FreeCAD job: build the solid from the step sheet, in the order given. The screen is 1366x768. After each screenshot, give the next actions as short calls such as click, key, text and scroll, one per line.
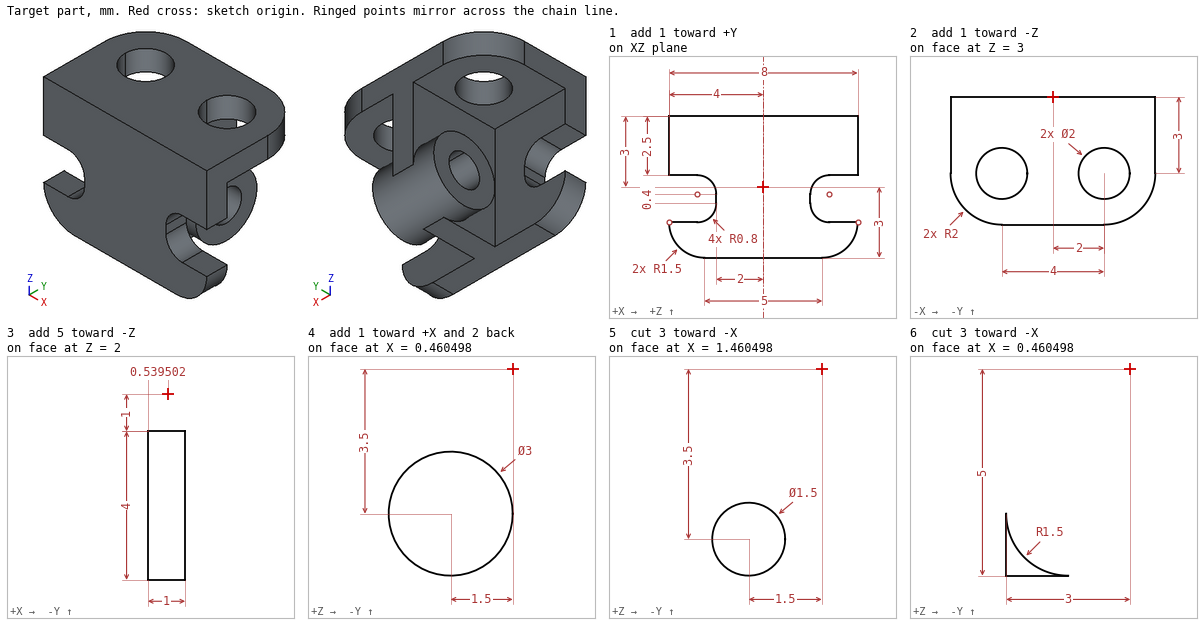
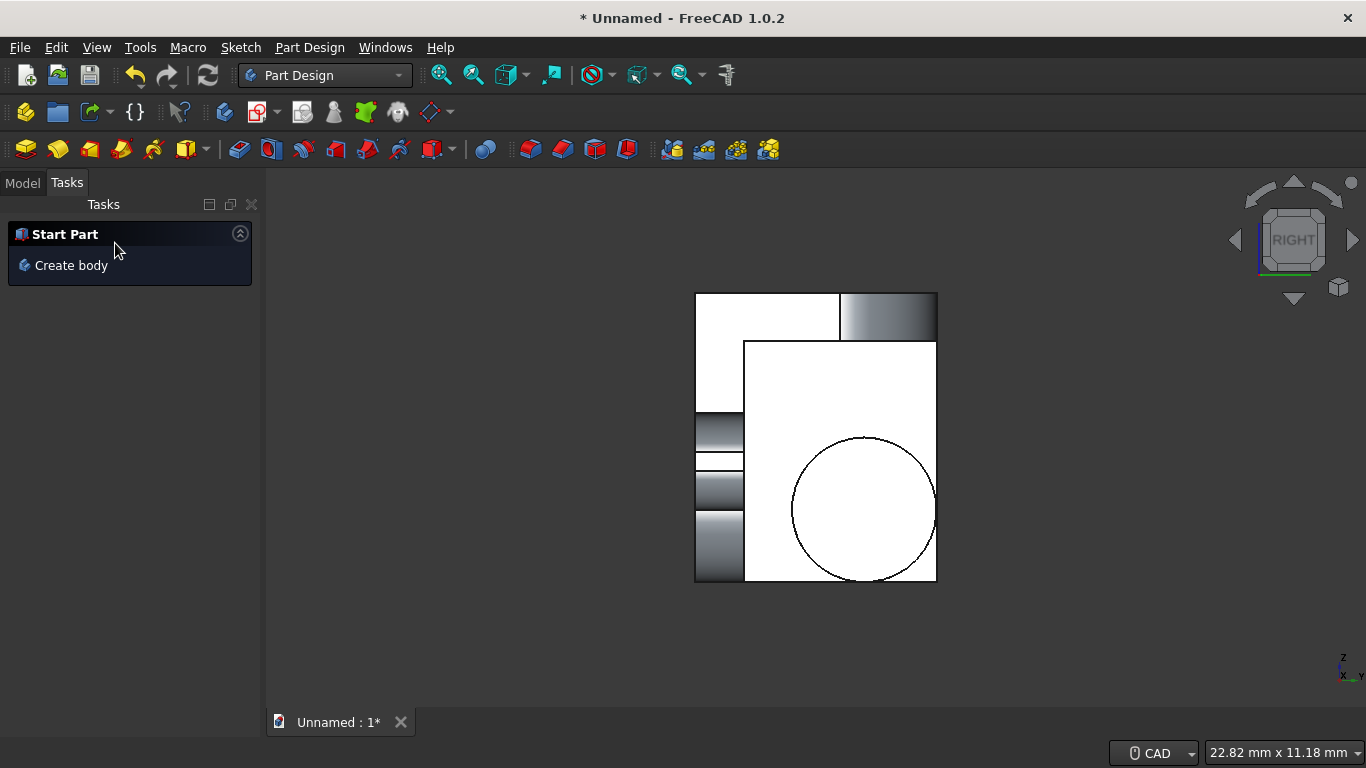
click(864, 509)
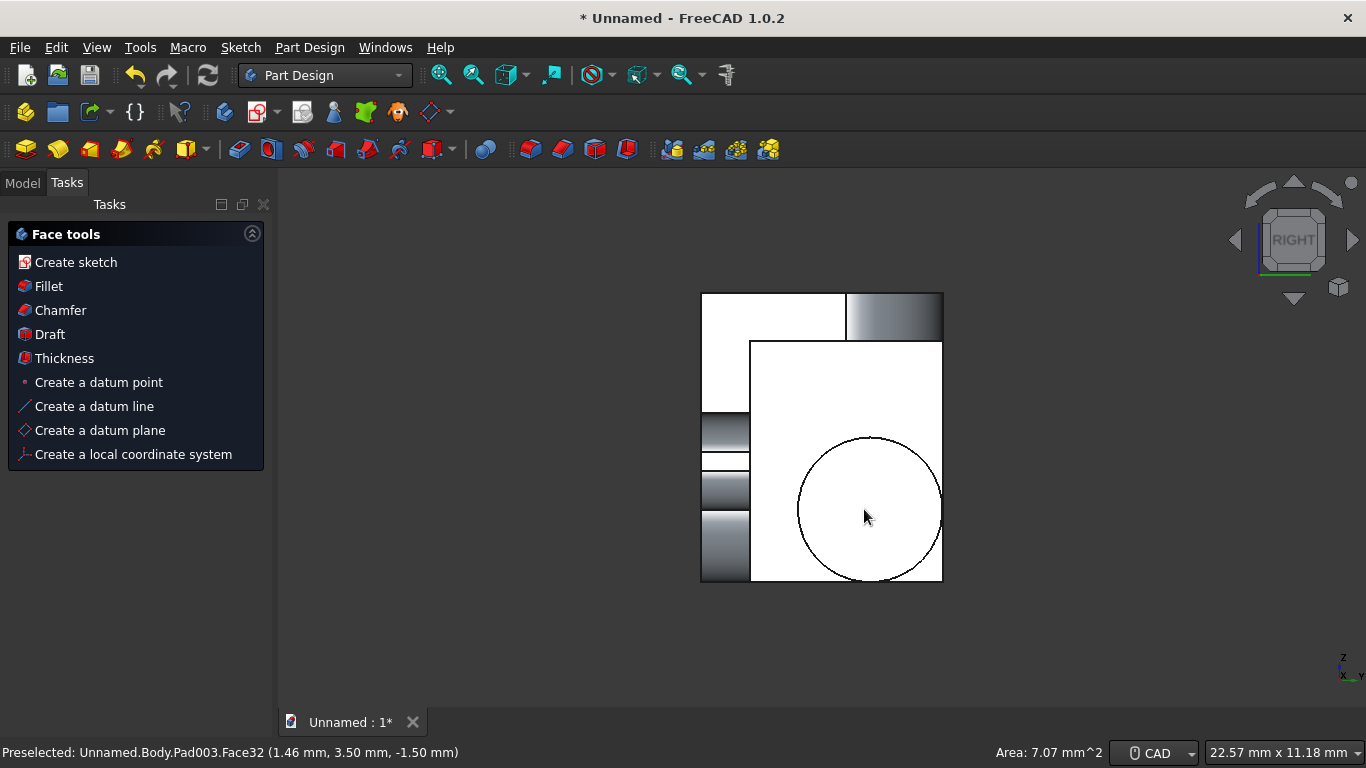
click(258, 112)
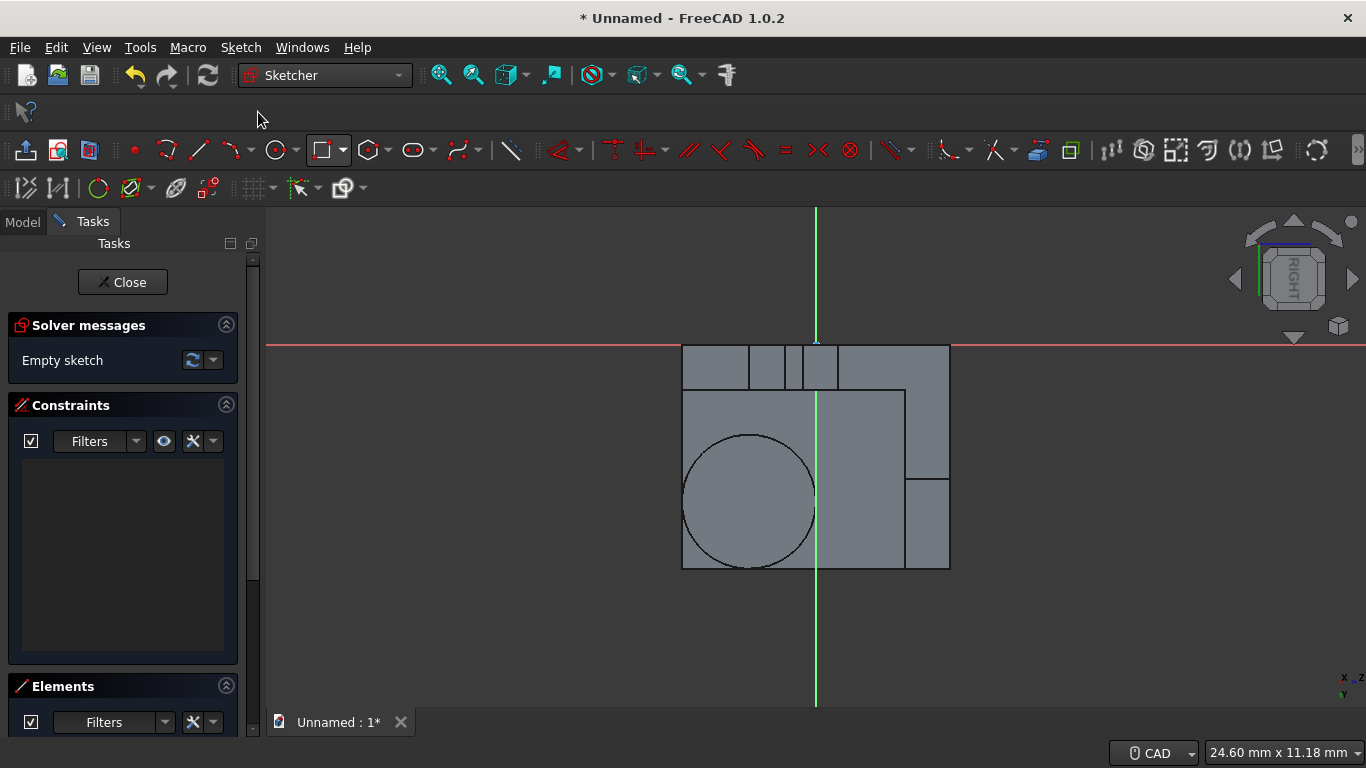
click(90, 150)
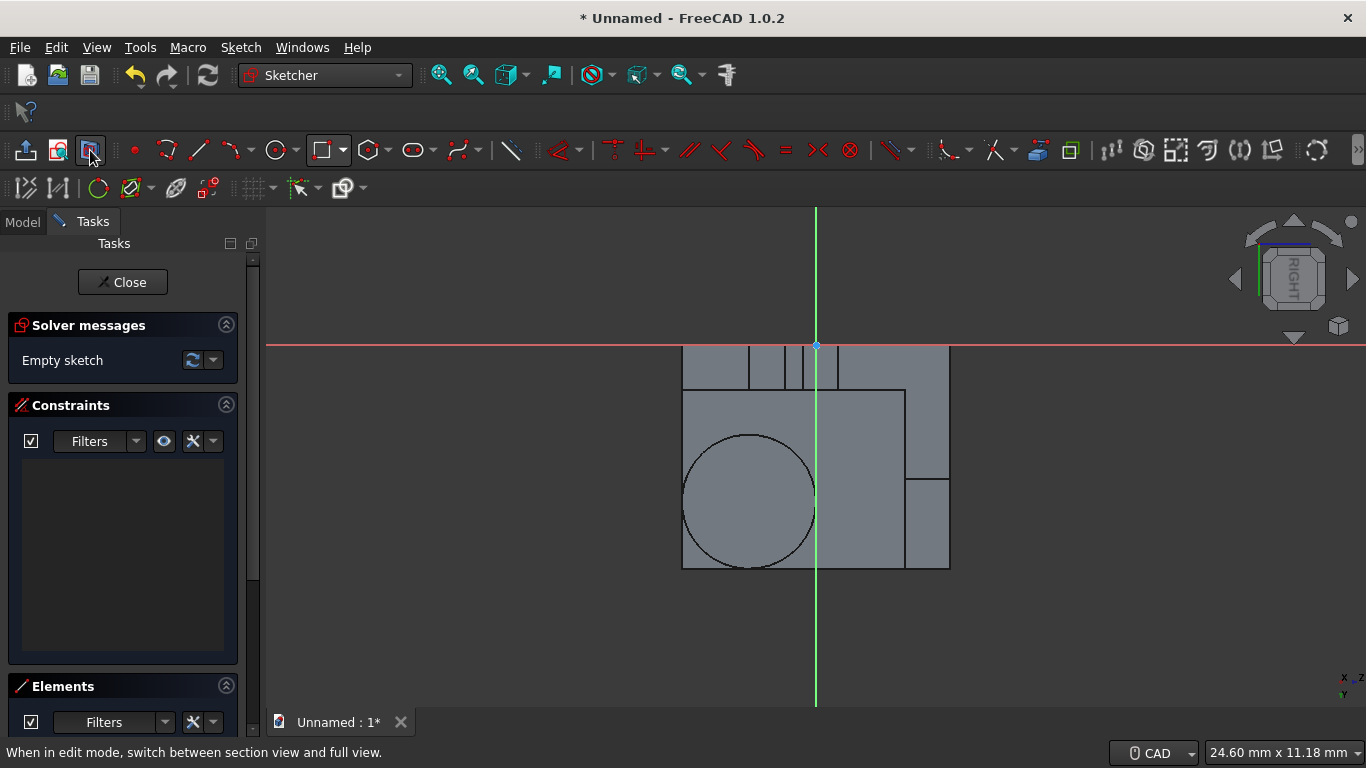
scroll(749, 513, up, 8)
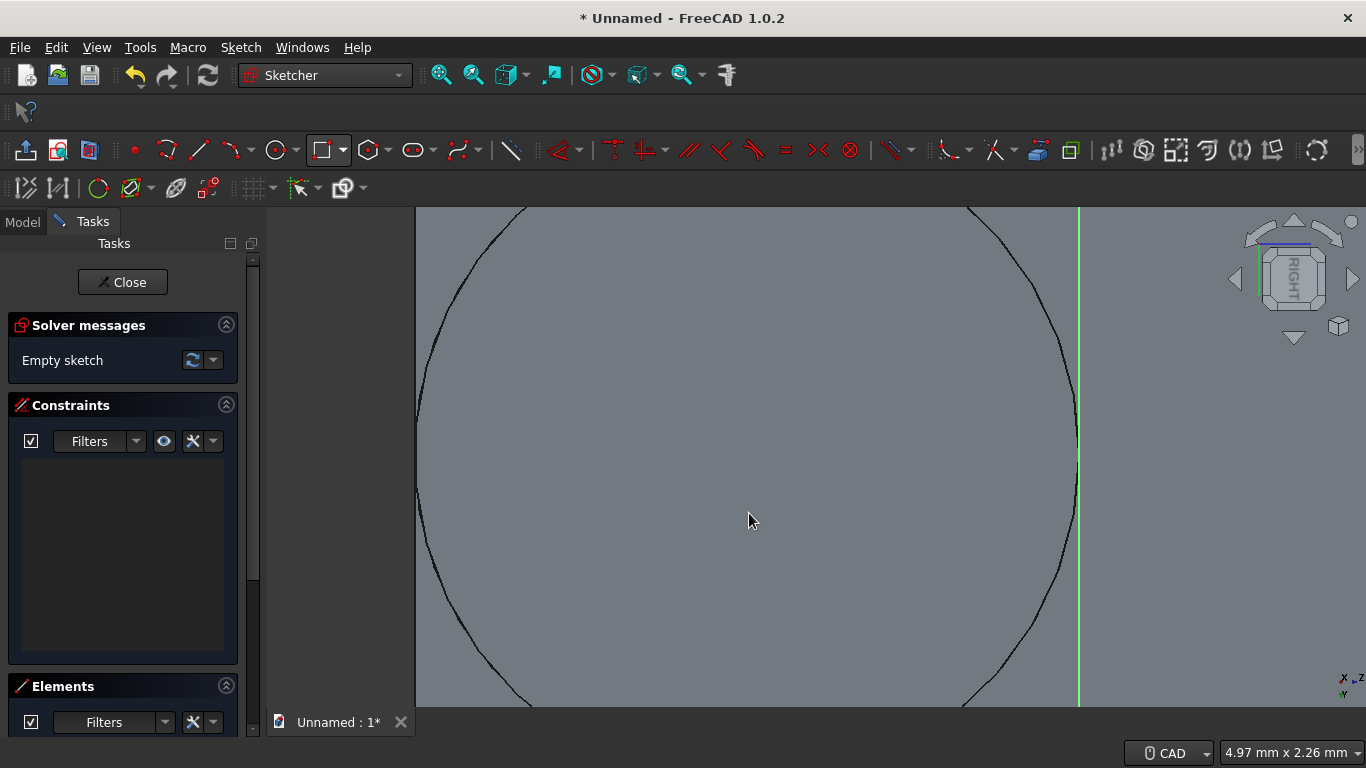
click(276, 150)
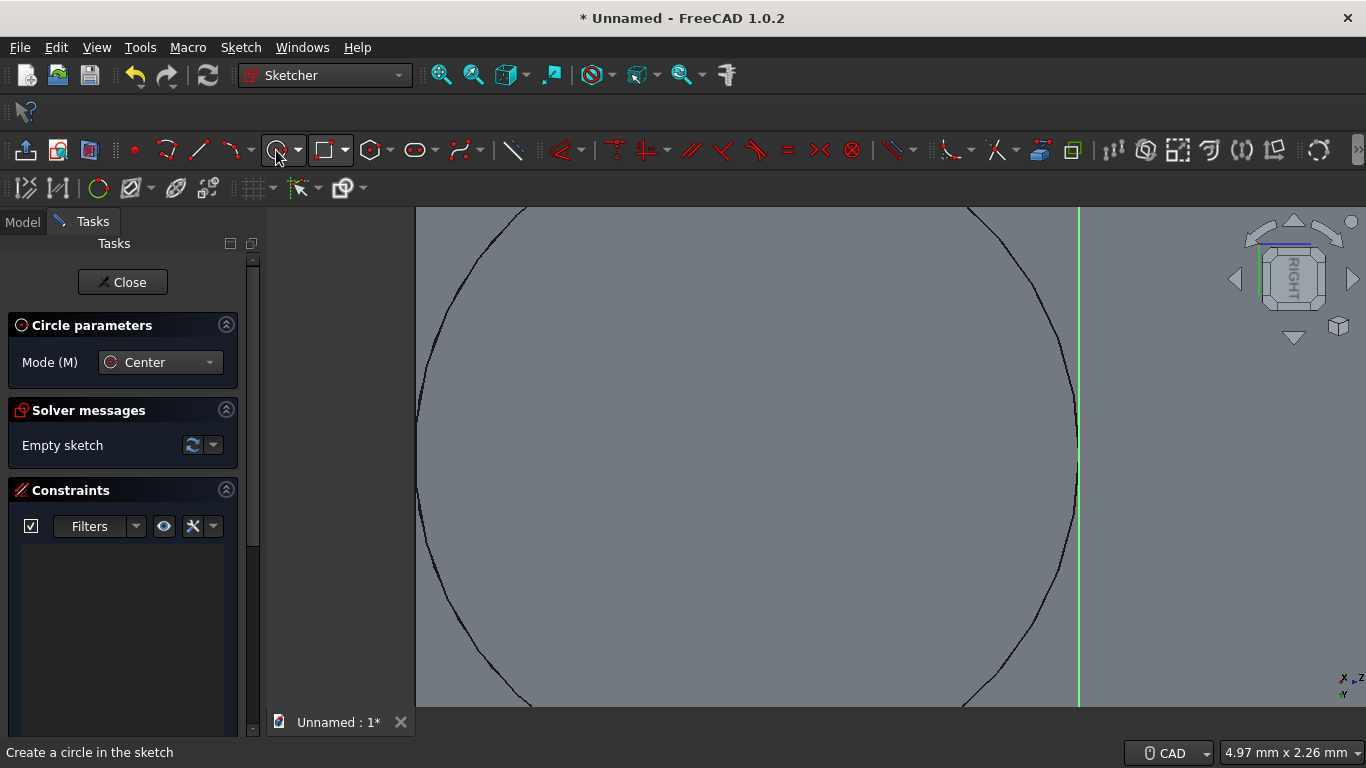
click(747, 455)
click(864, 337)
key(Escape)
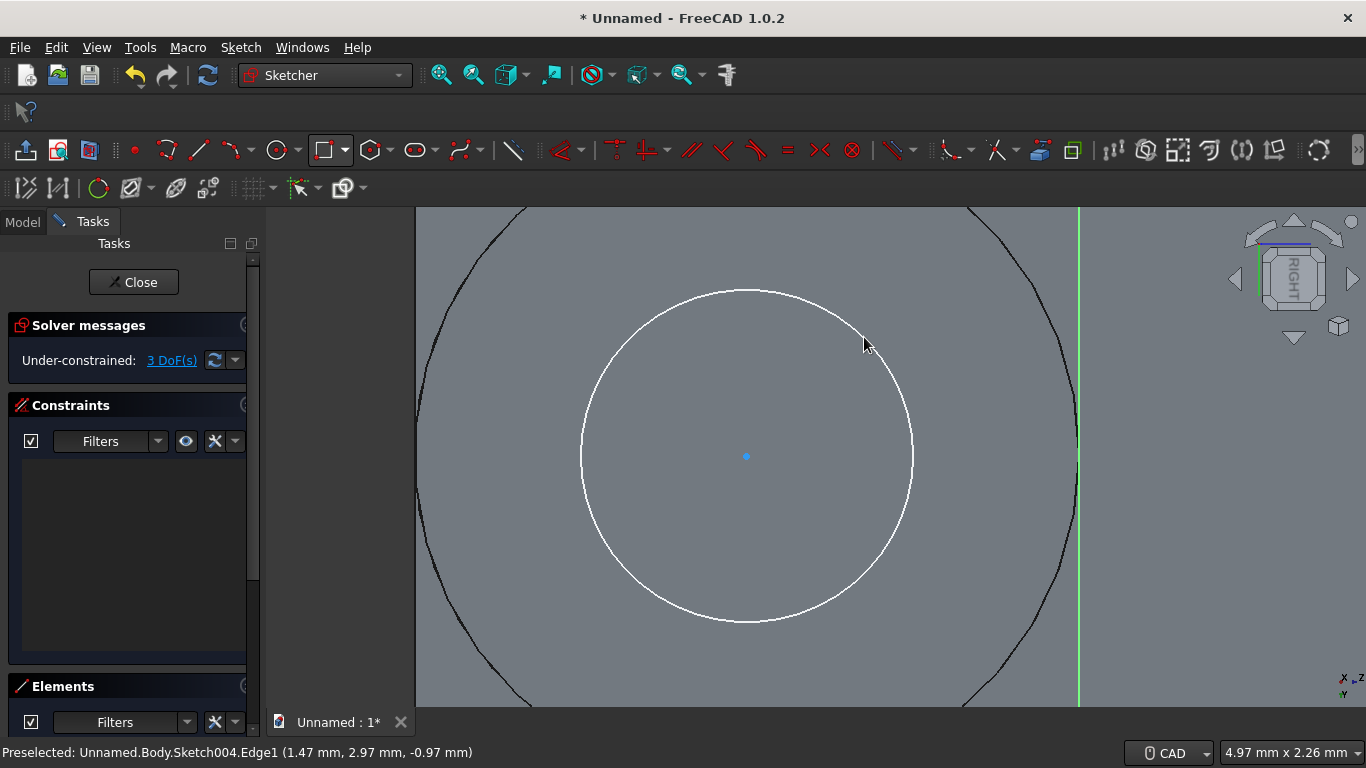
click(560, 150)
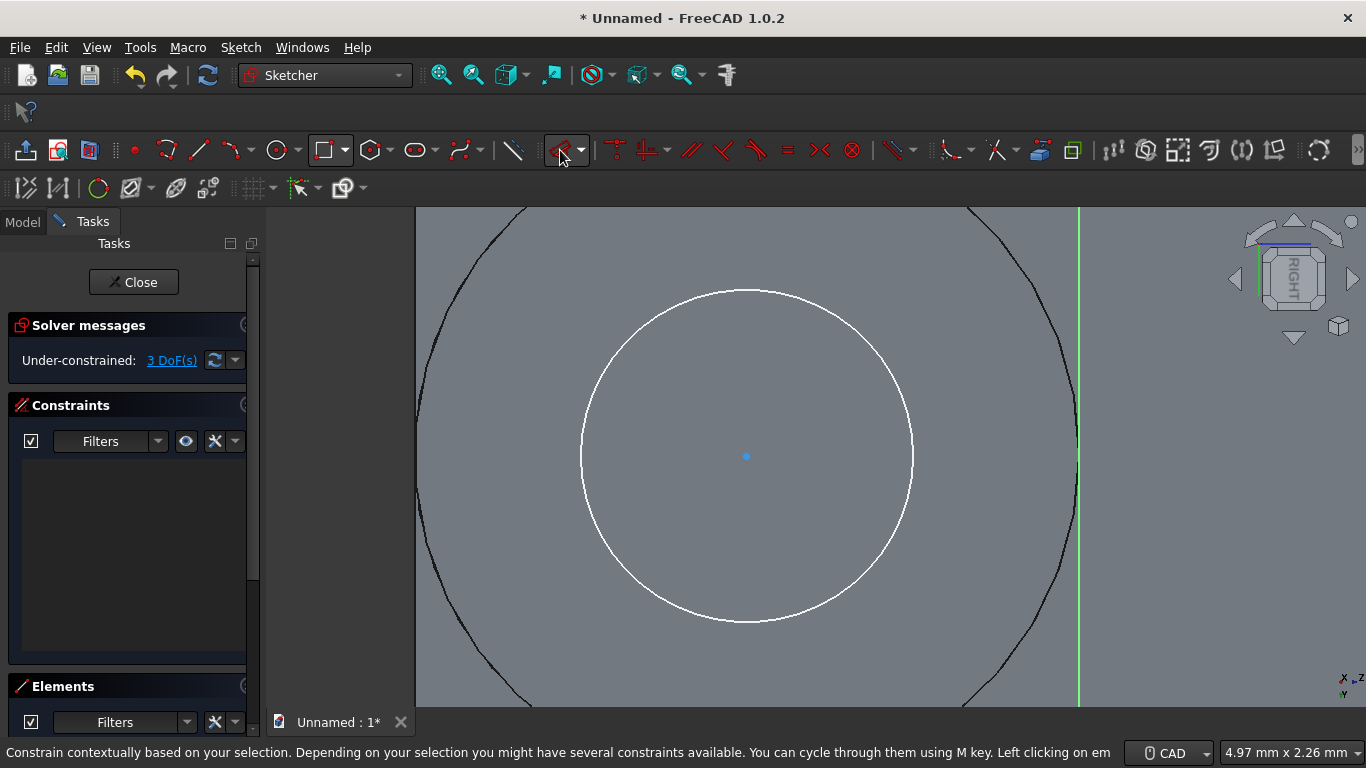
click(864, 338)
click(887, 315)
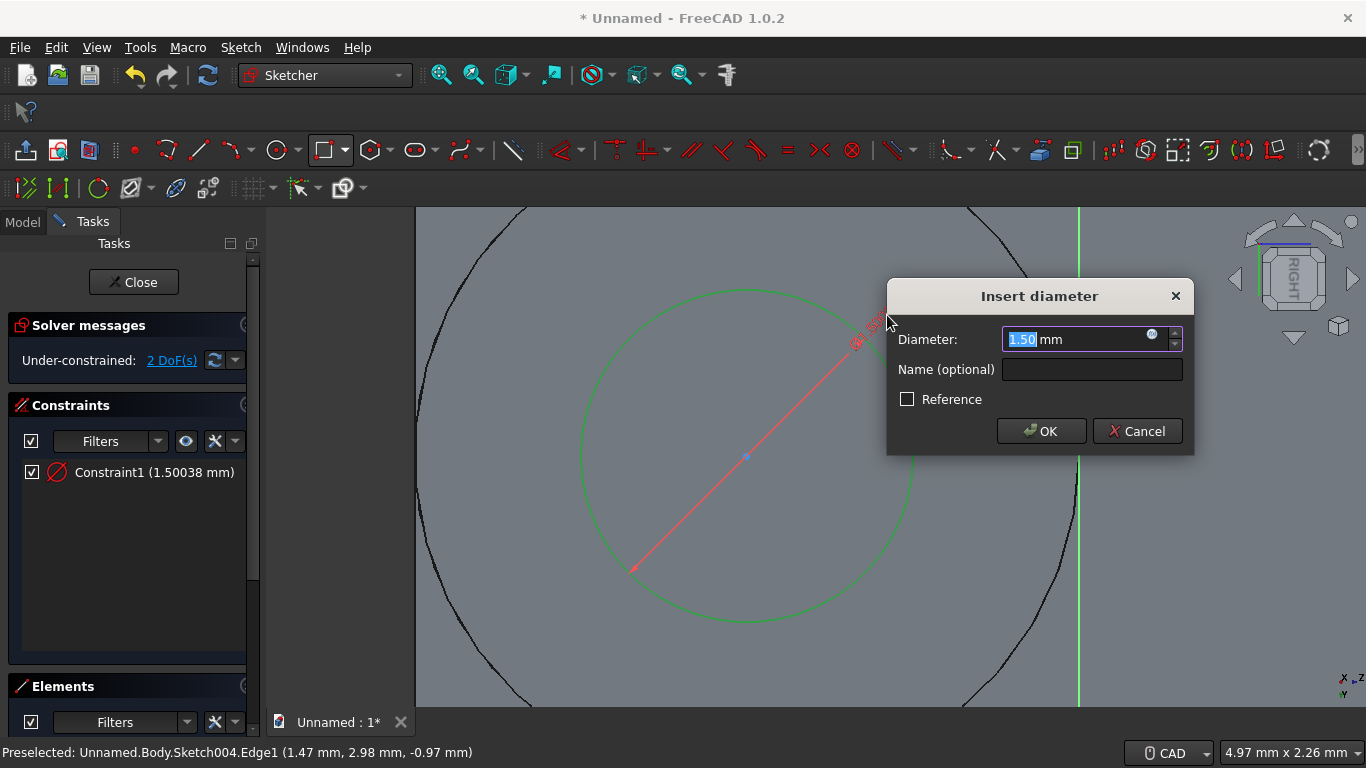
text(1.5)
key(Return)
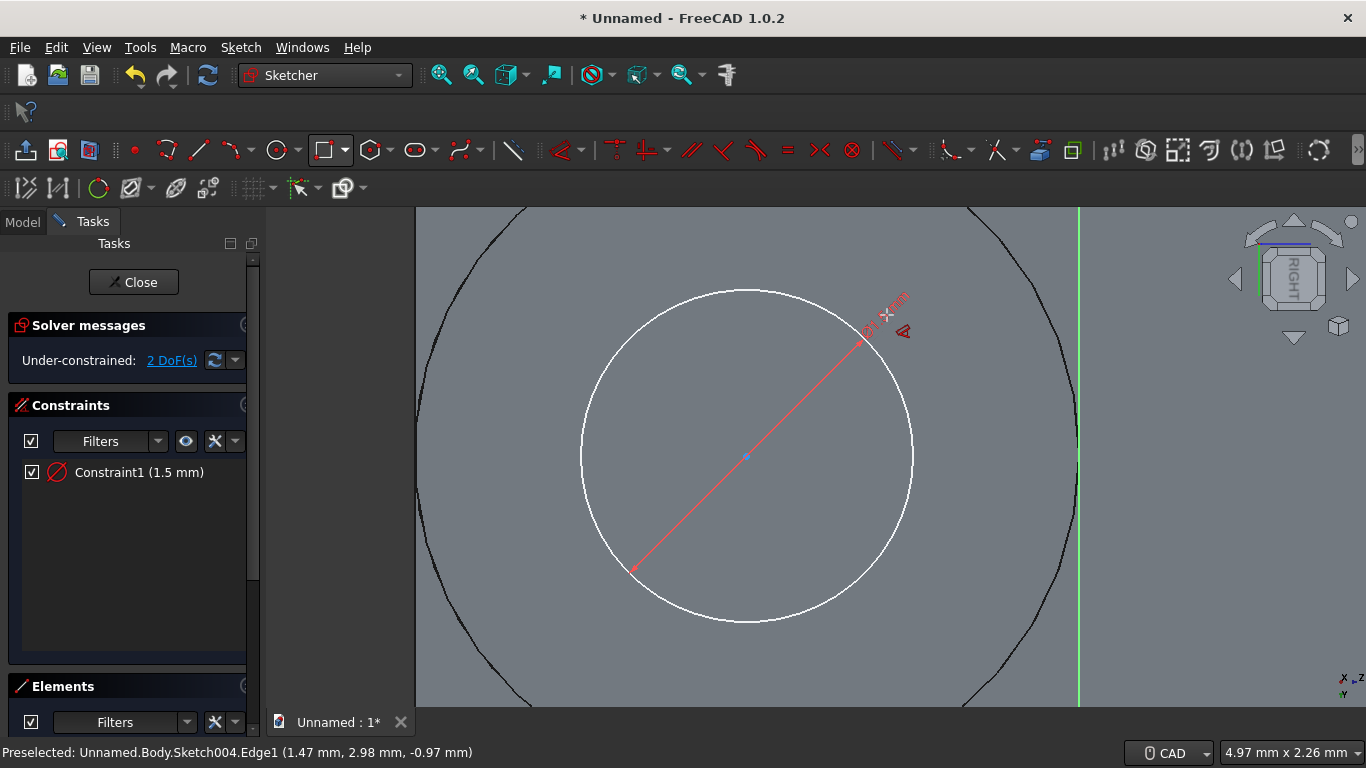
click(747, 456)
click(837, 490)